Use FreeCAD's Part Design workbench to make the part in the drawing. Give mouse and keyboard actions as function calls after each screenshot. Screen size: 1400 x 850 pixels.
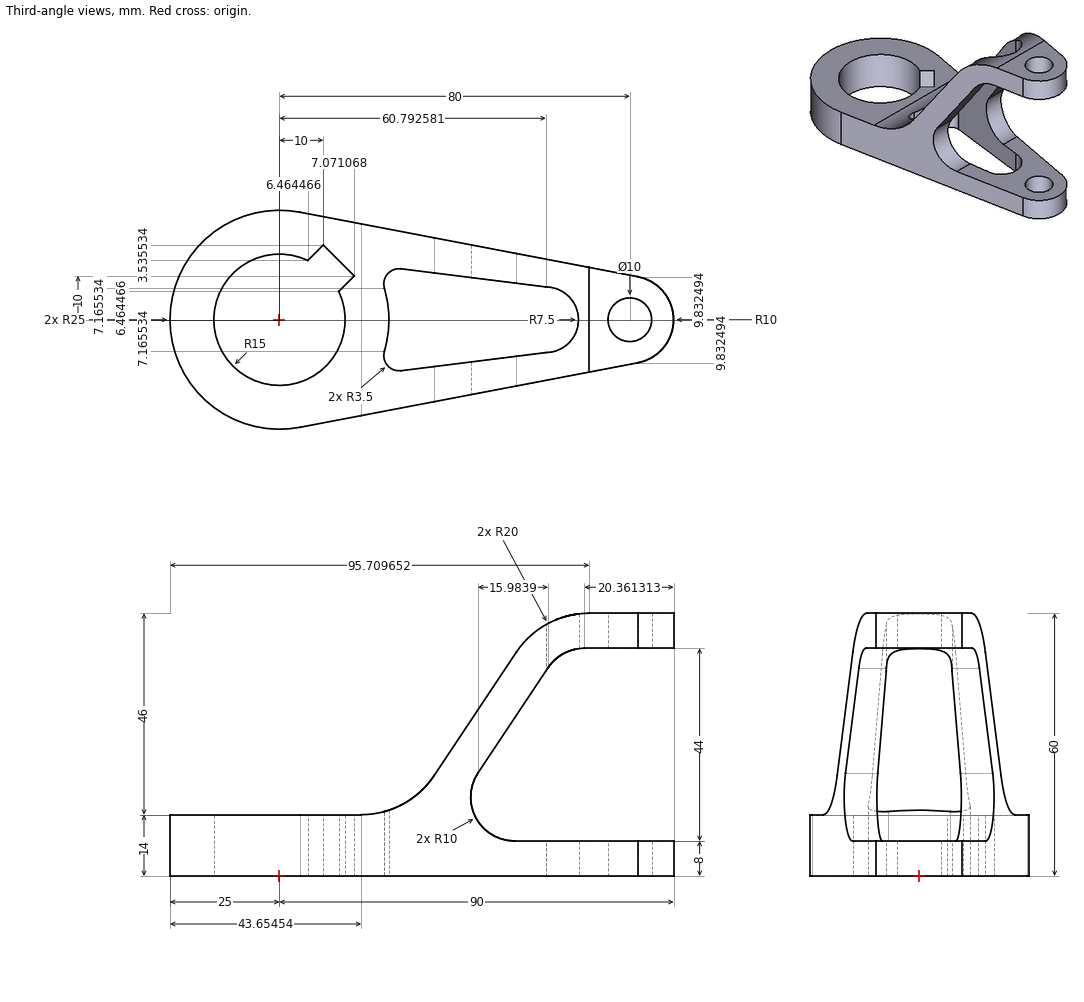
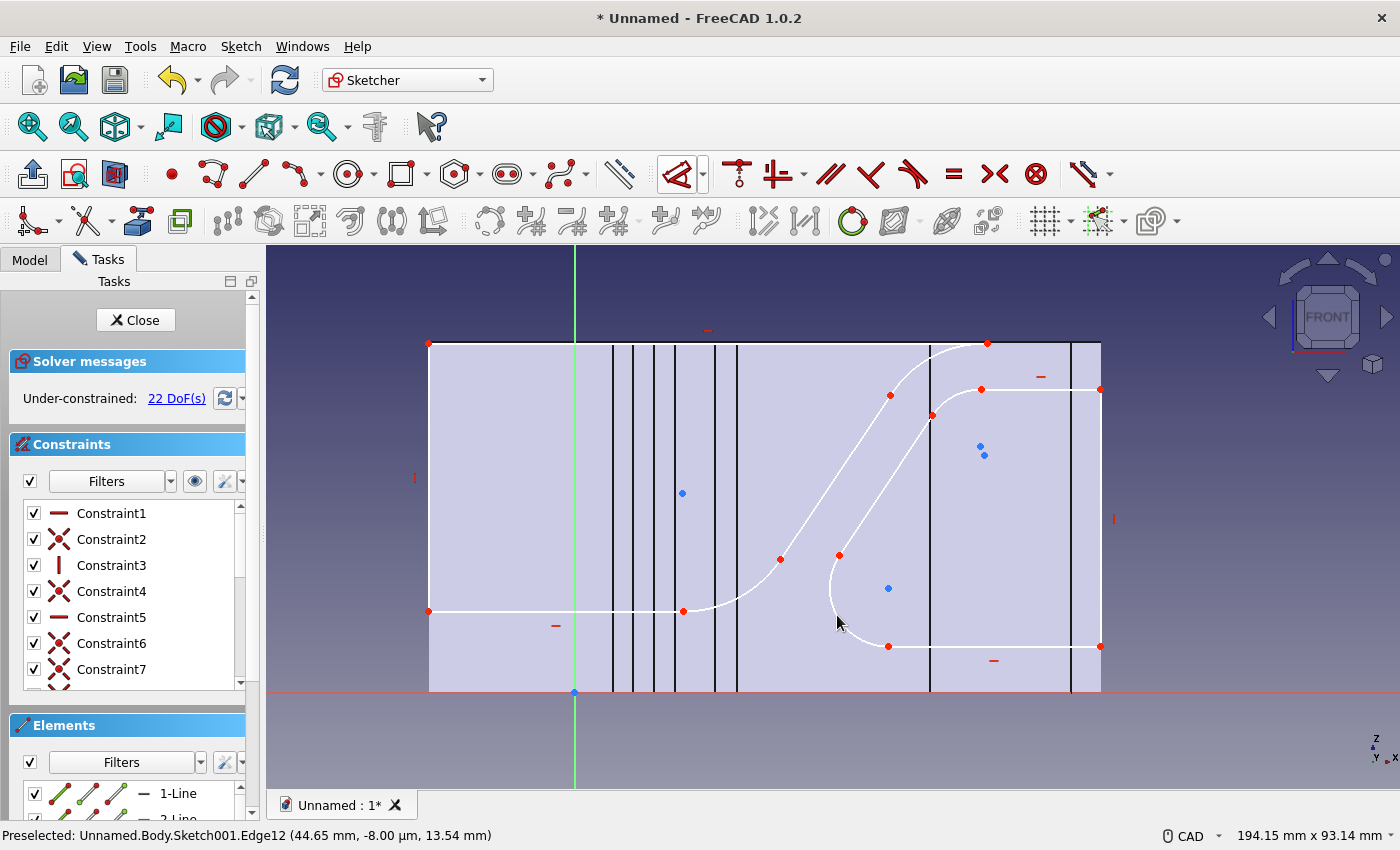
click(607, 612)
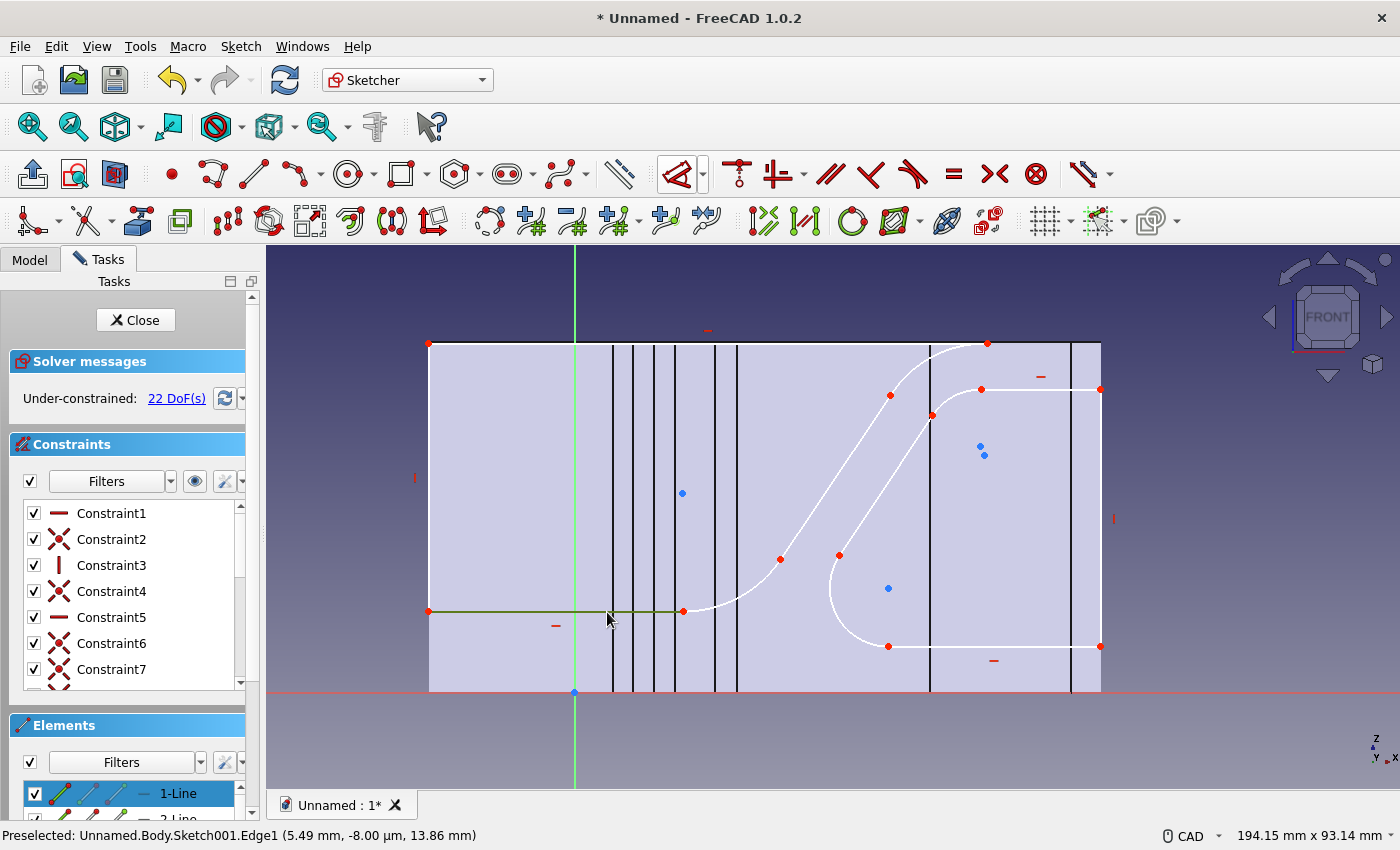
click(717, 606)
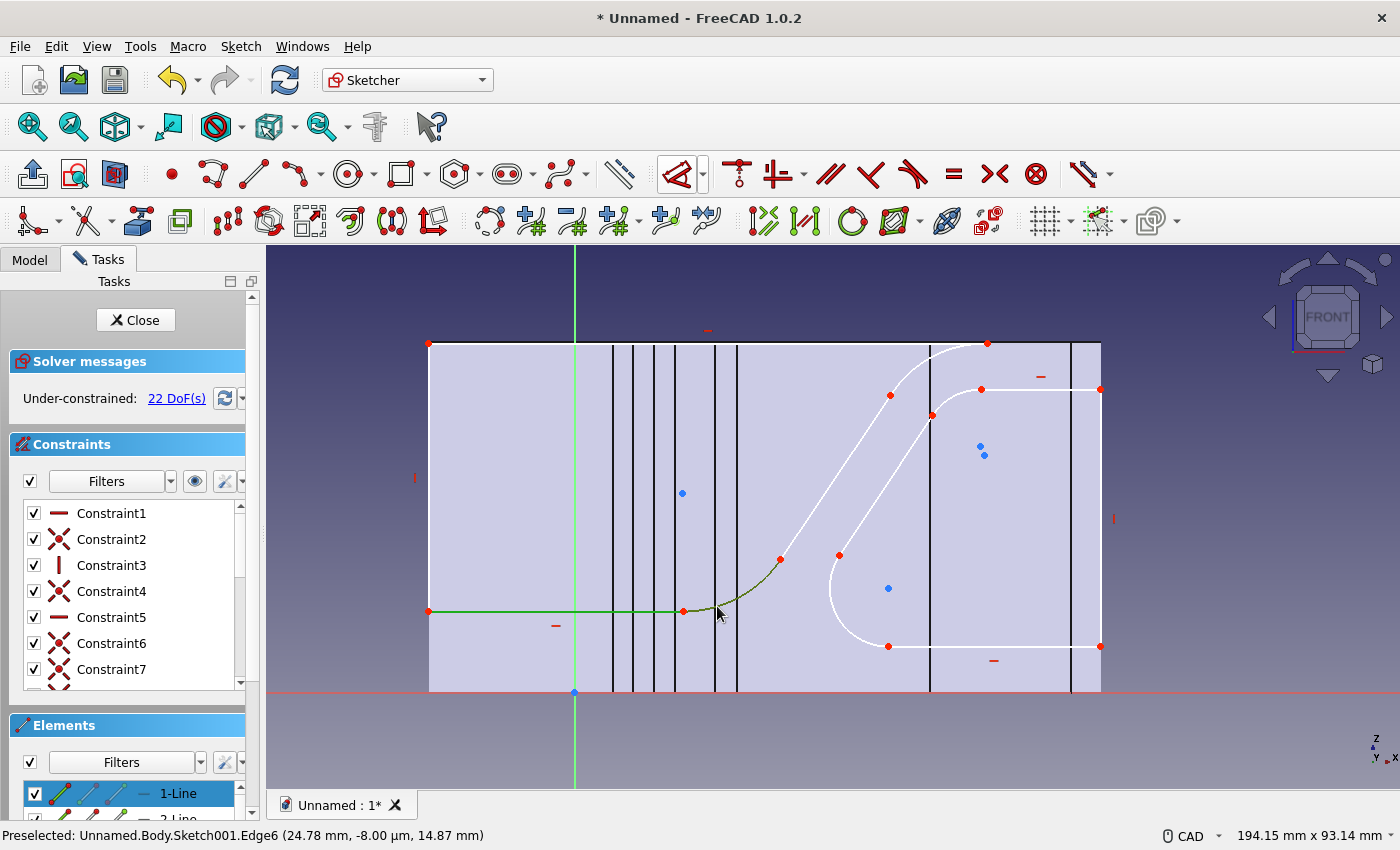
click(913, 174)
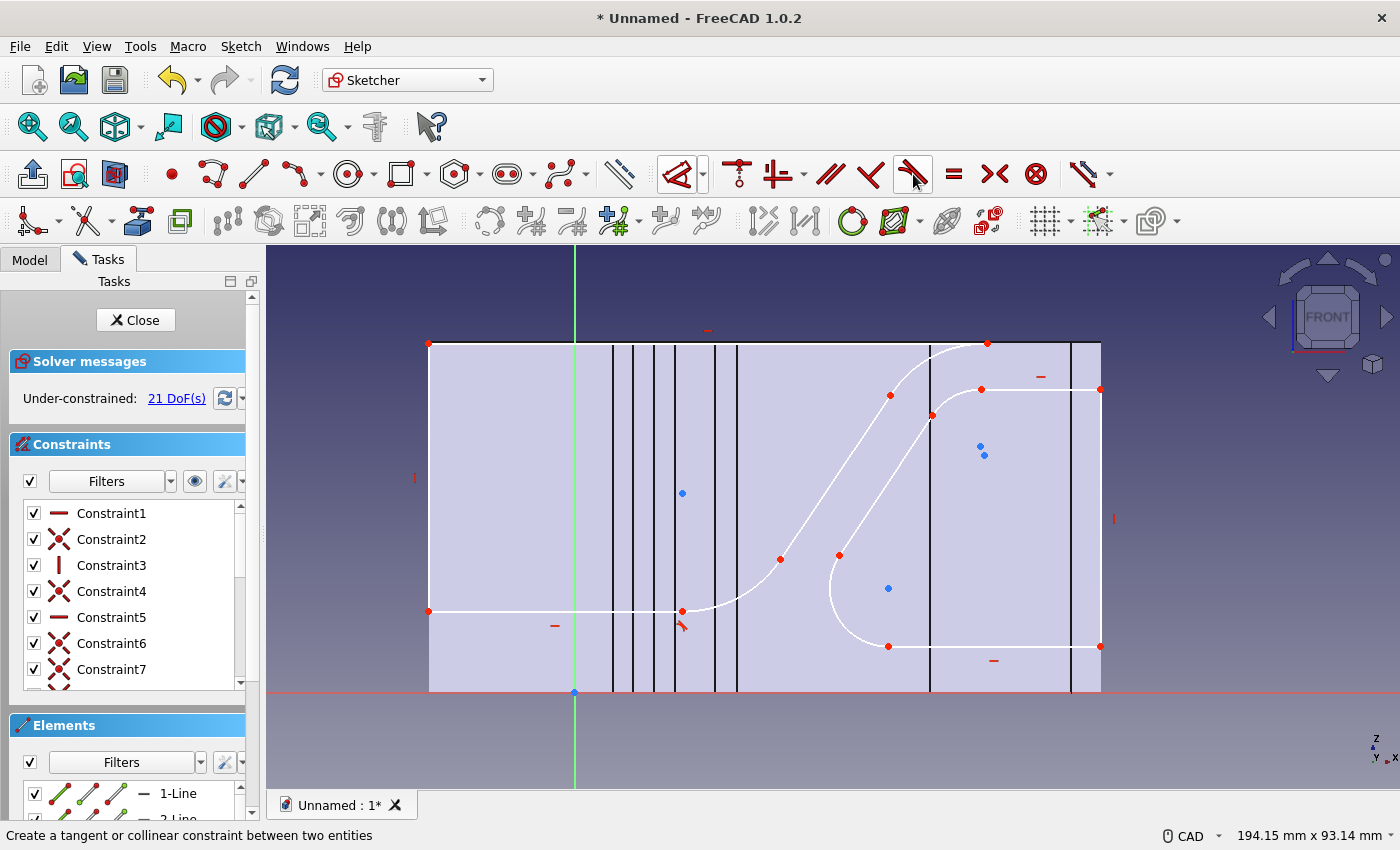
click(596, 344)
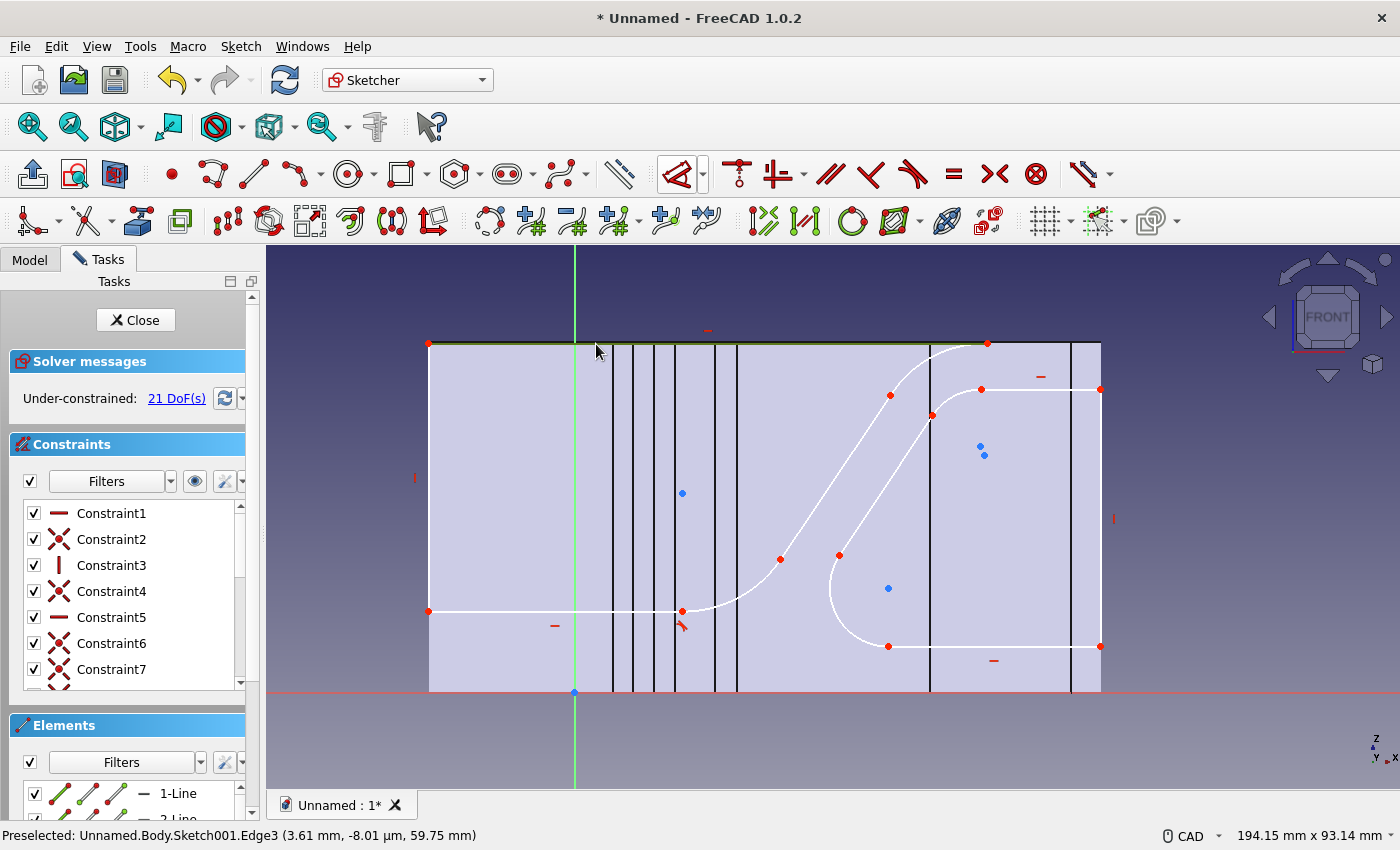
click(913, 370)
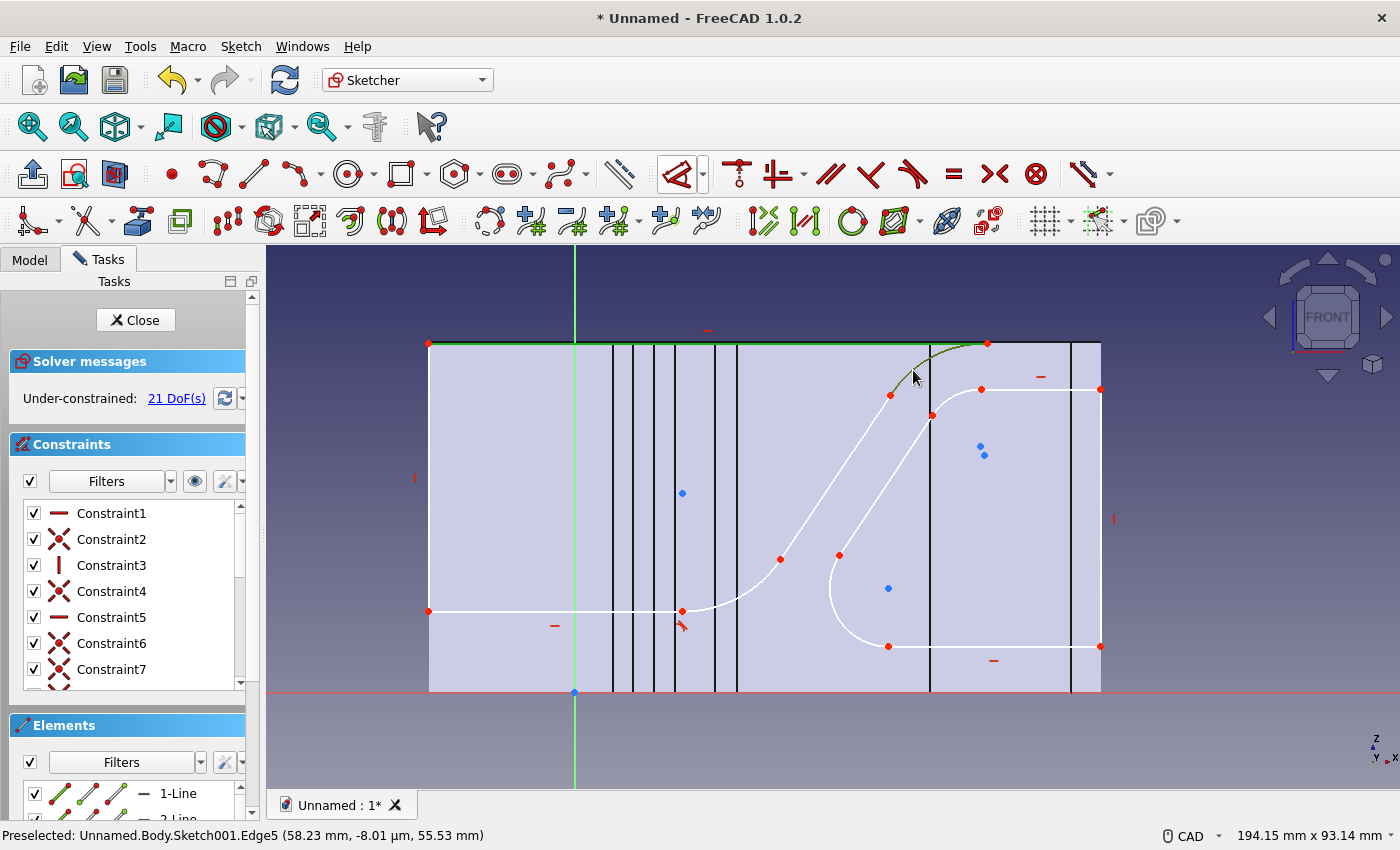
click(913, 174)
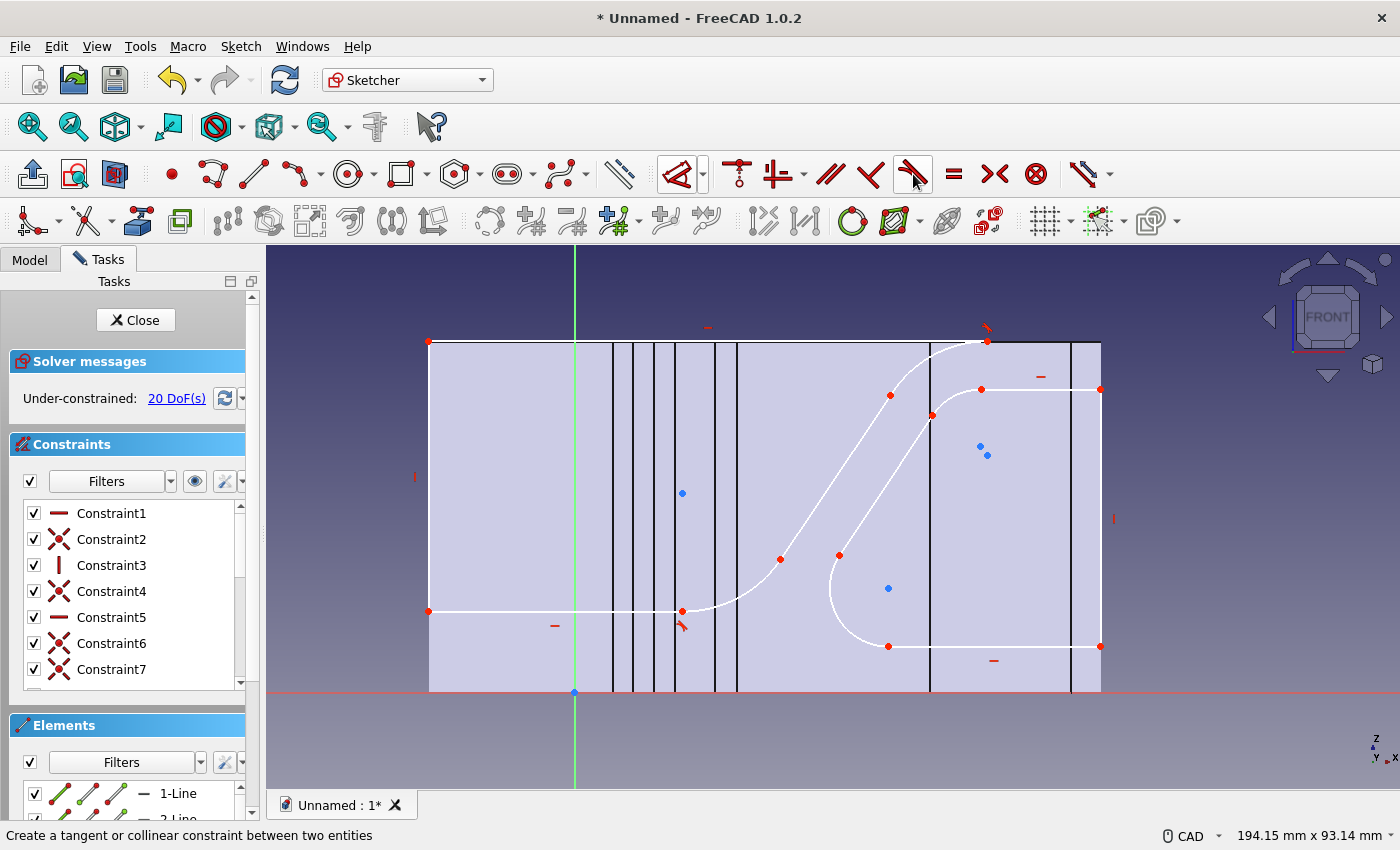
click(858, 445)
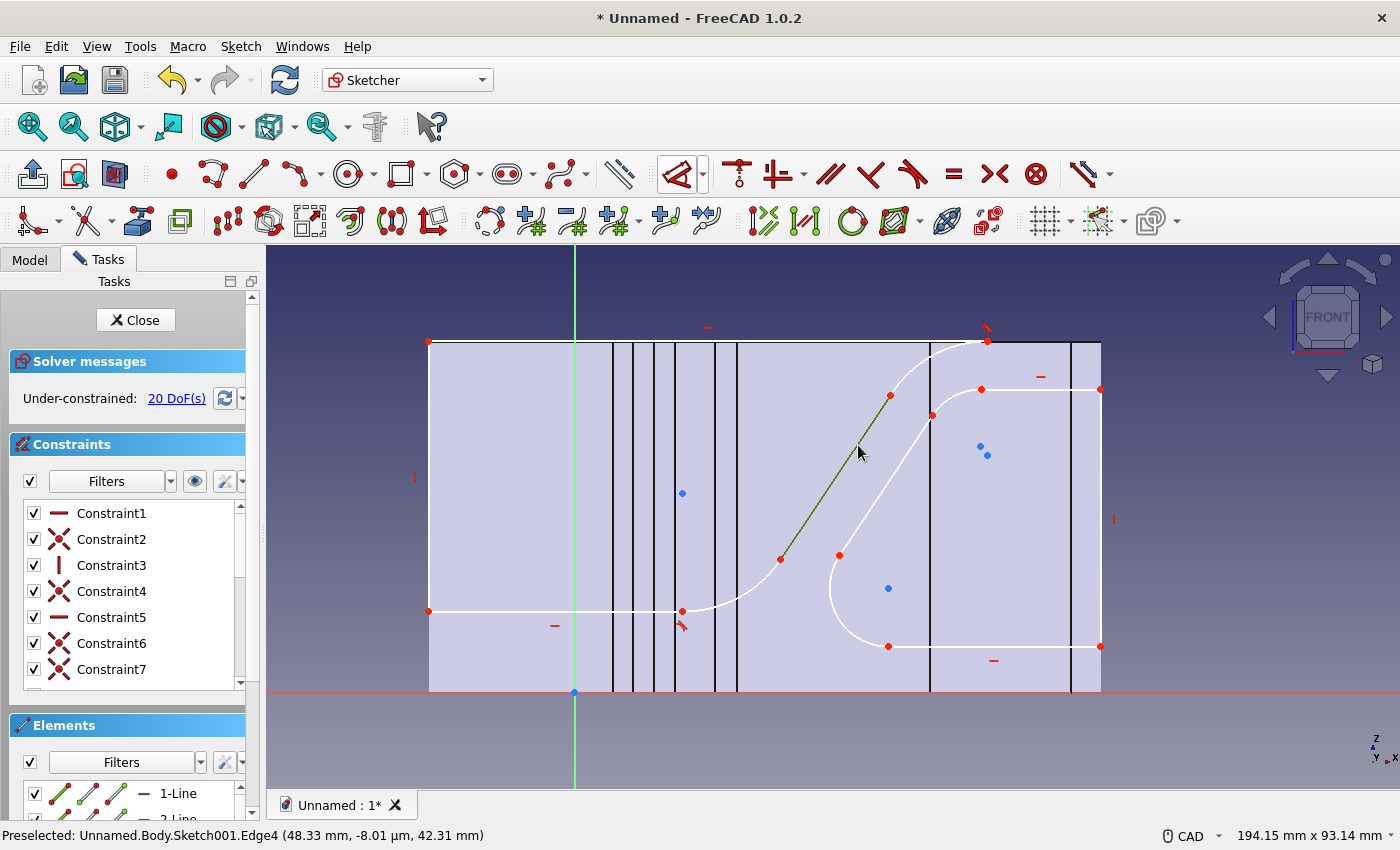
click(913, 369)